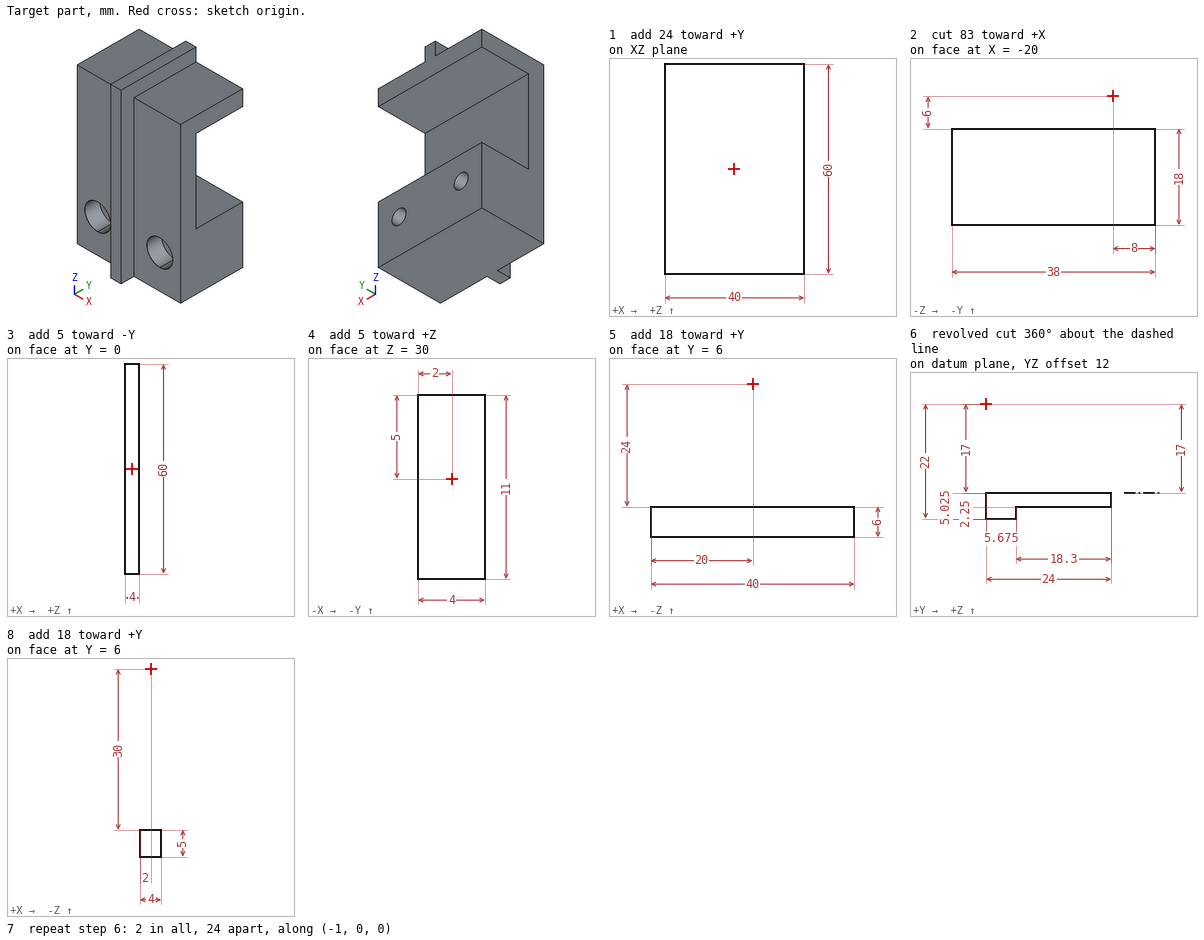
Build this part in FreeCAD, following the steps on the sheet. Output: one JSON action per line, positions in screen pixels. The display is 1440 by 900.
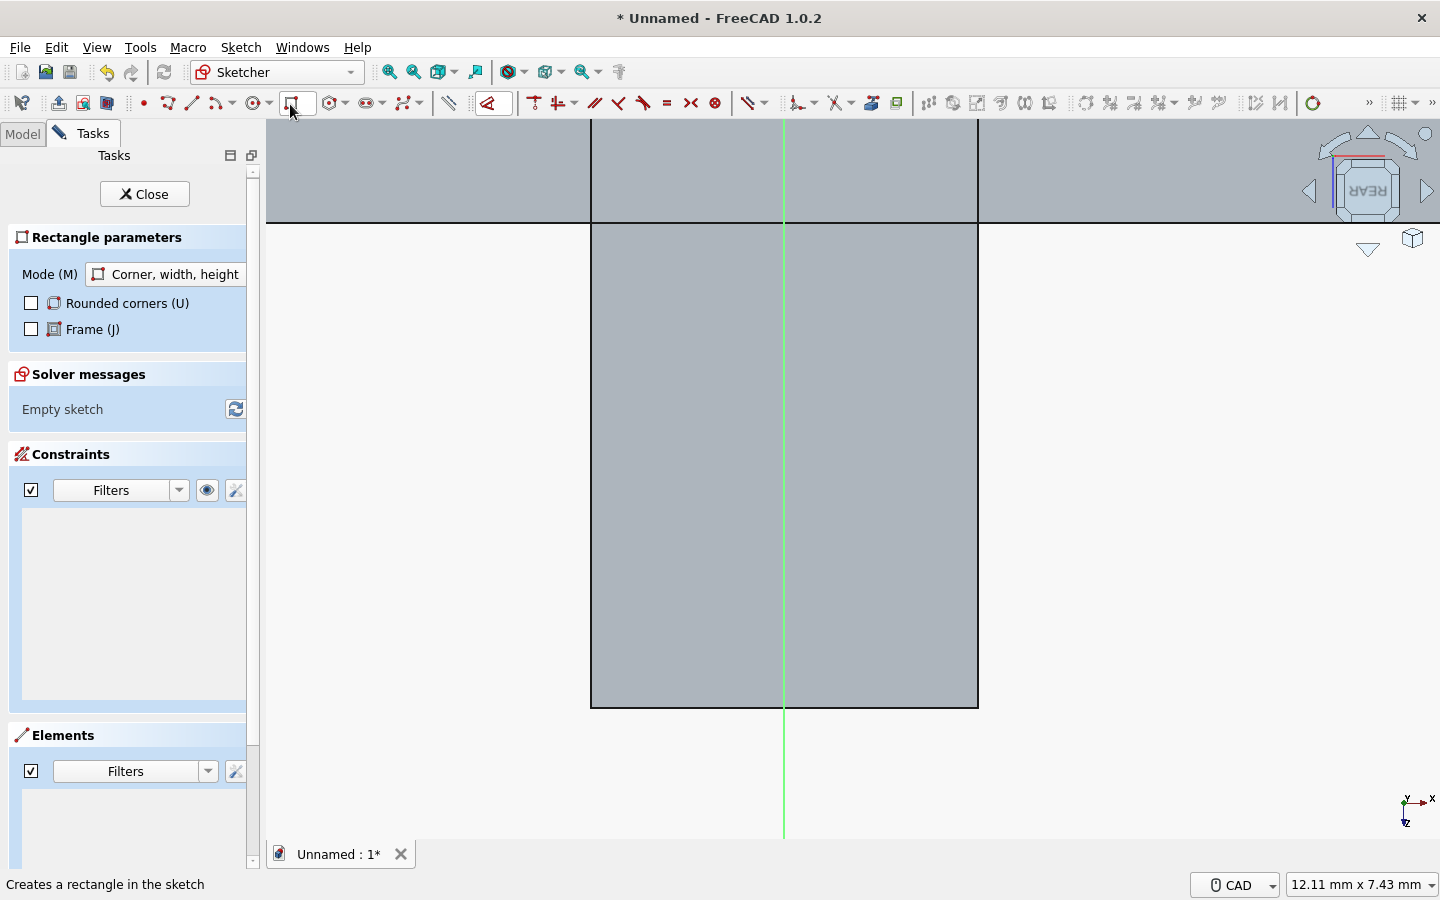
{"action": "left_click", "coordinate": [591, 223]}
{"action": "mouse_move", "coordinate": [978, 708]}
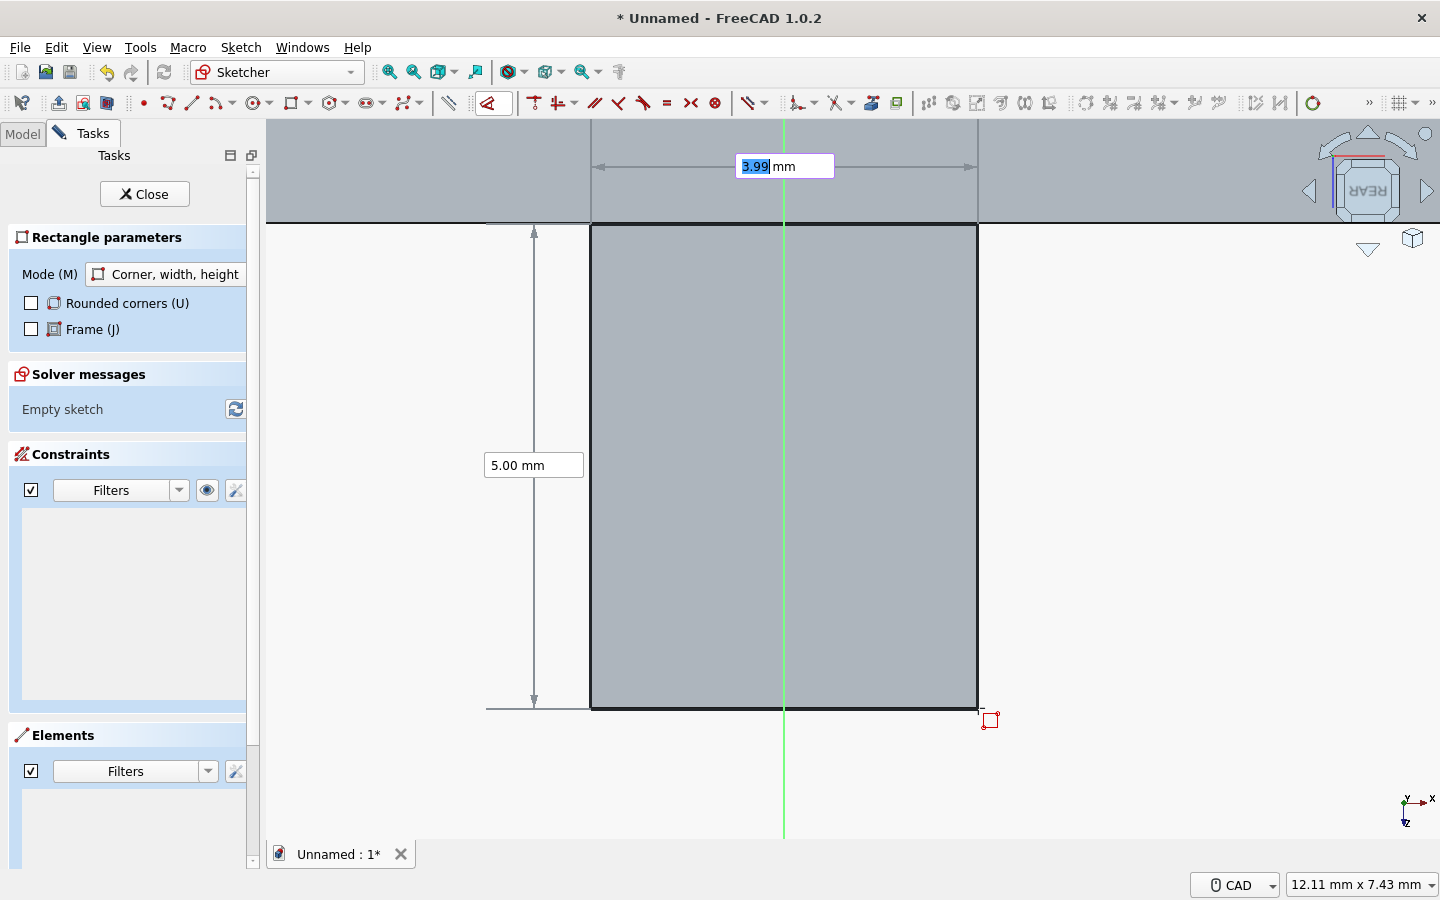
{"action": "type", "text": "4"}
{"action": "key", "text": "Tab"}
{"action": "type", "text": "5"}
{"action": "key", "text": "Return"}
{"action": "key", "text": "Escape"}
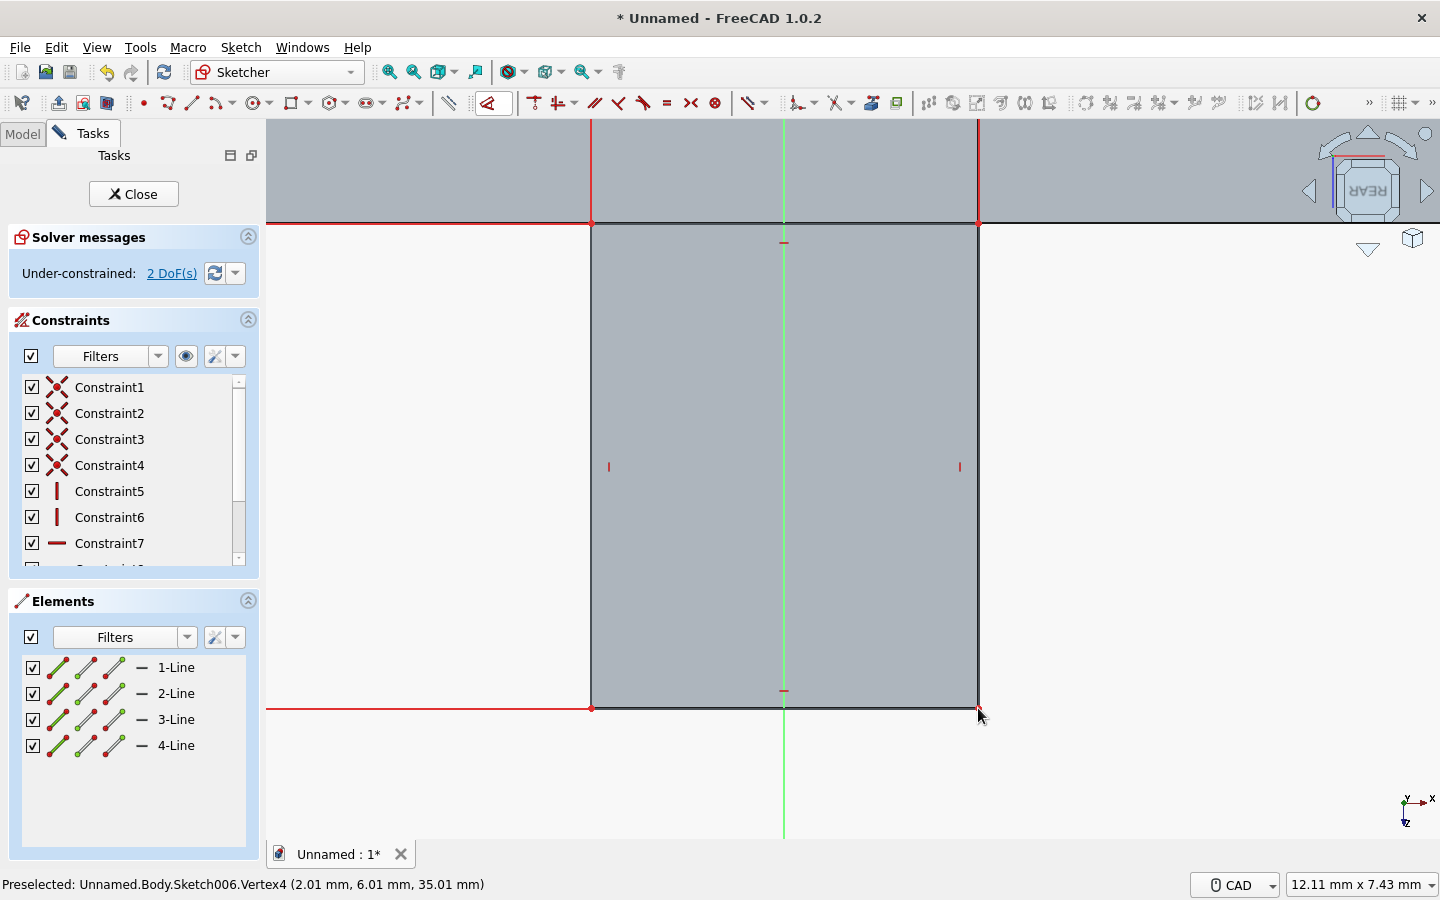
{"action": "key", "text": "d"}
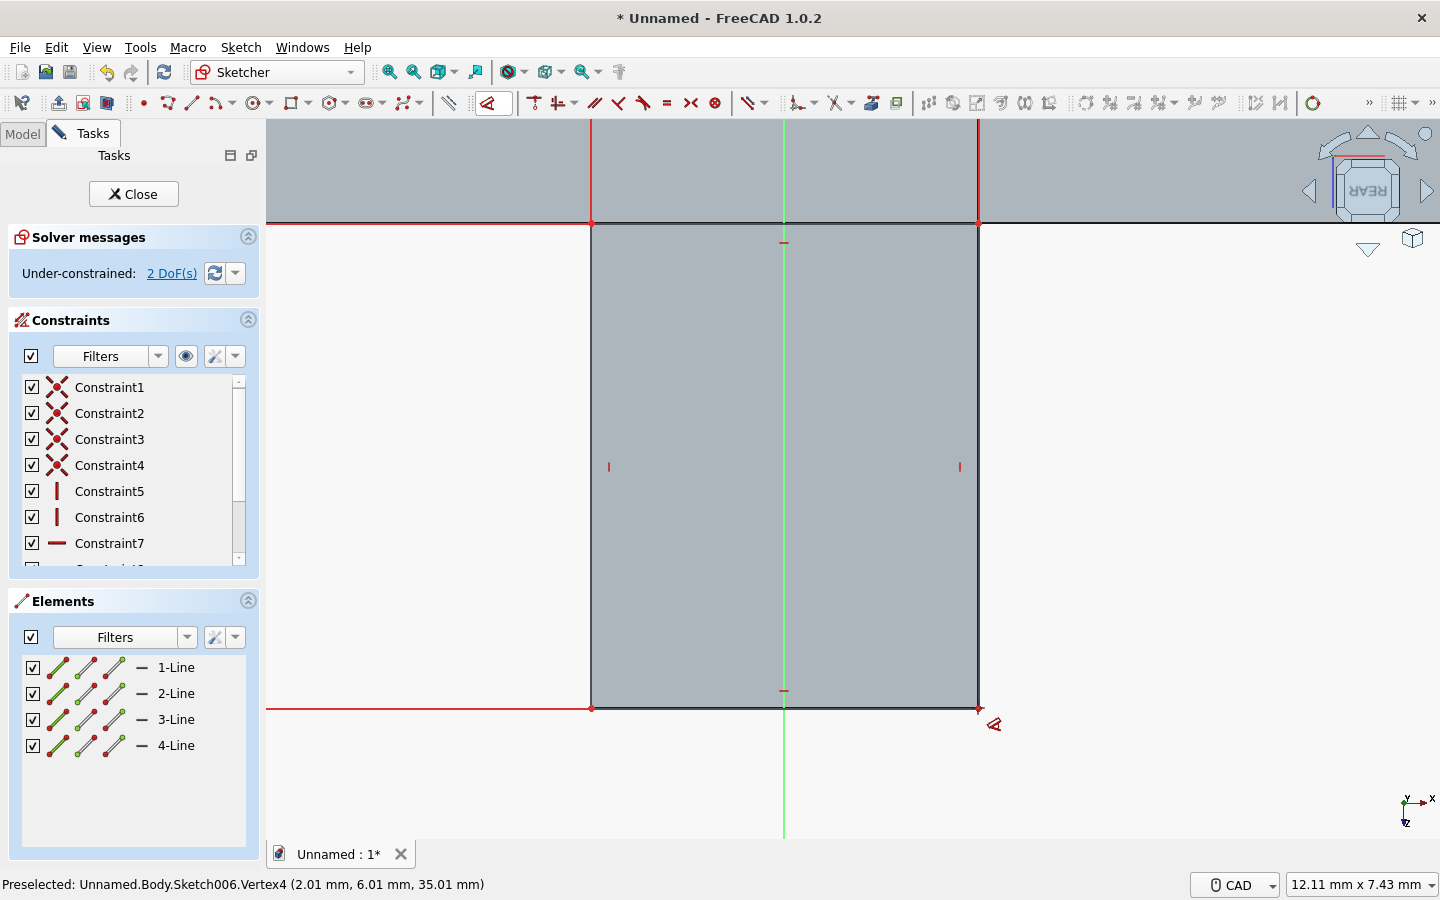
{"action": "left_click", "coordinate": [591, 224]}
{"action": "left_click", "coordinate": [688, 258]}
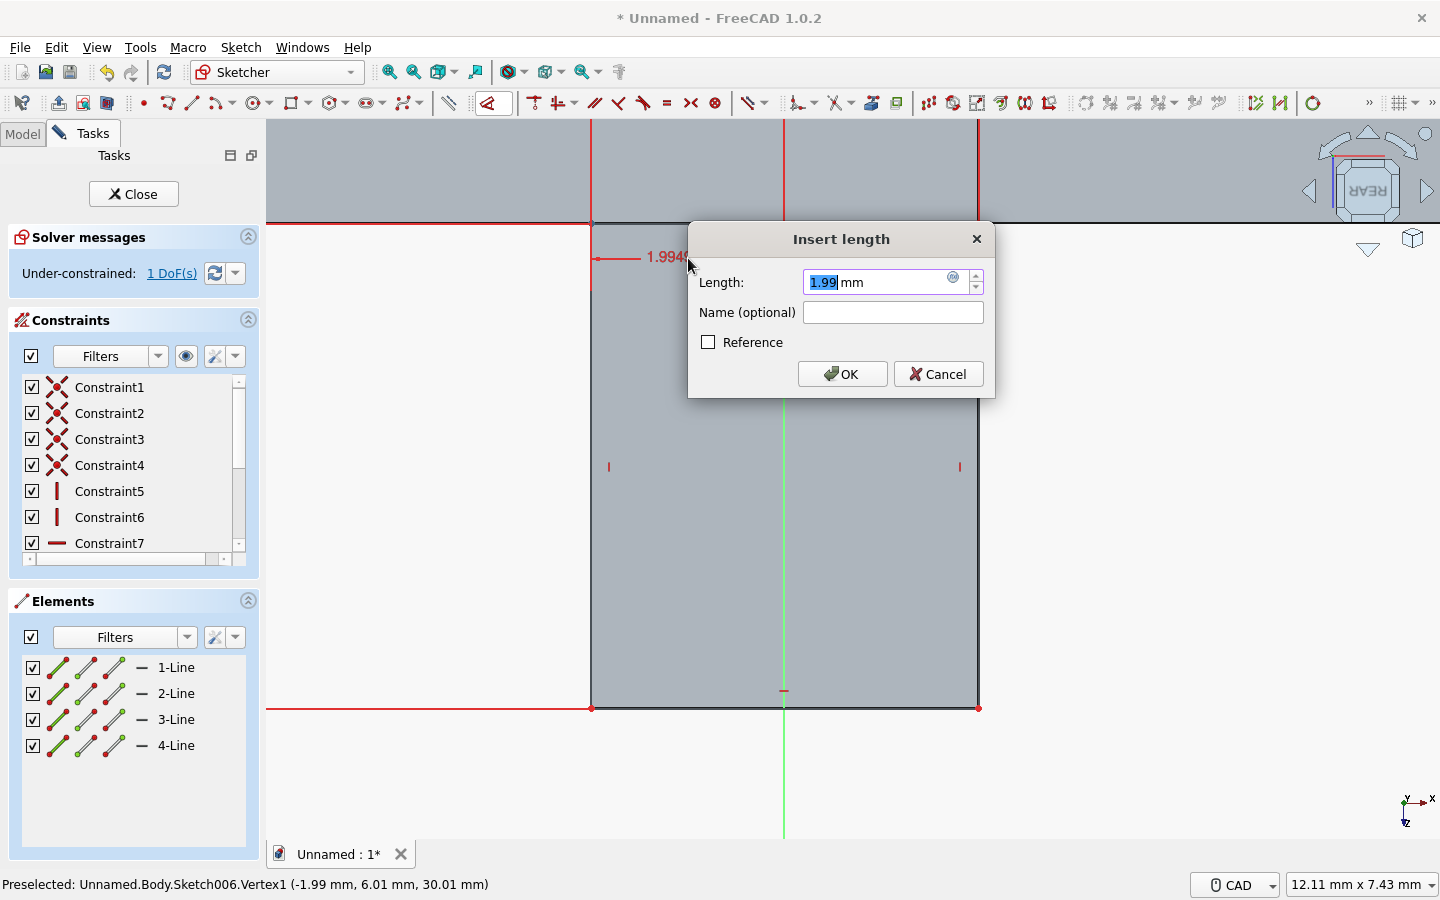
{"action": "type", "text": "2"}
{"action": "key", "text": "Return"}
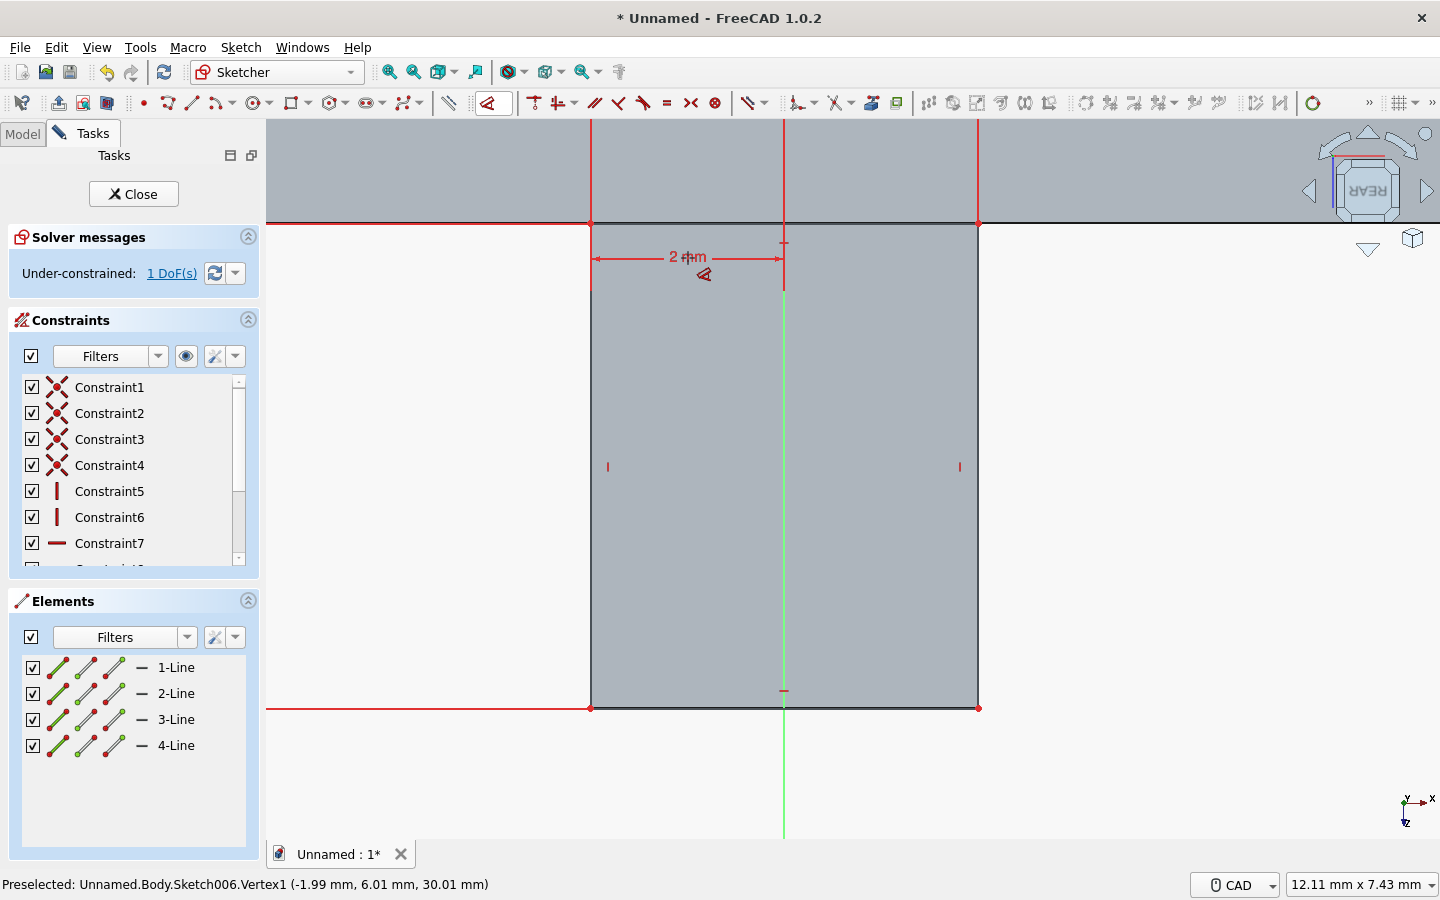
{"action": "left_click", "coordinate": [591, 224]}
{"action": "left_click", "coordinate": [557, 185]}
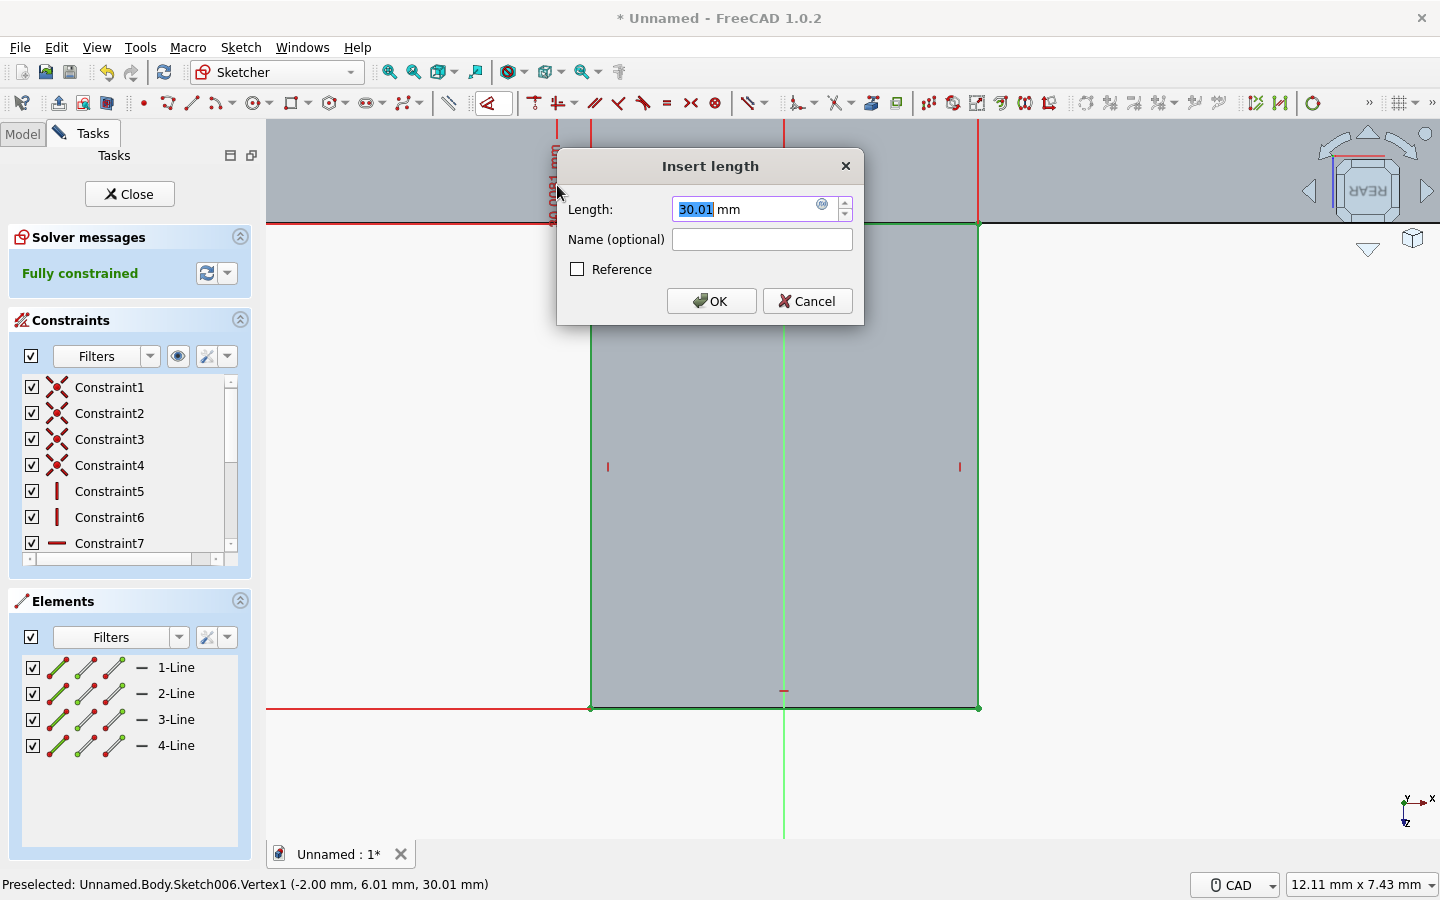
{"action": "type", "text": "30"}
{"action": "key", "text": "Return"}
{"action": "key", "text": "Escape"}